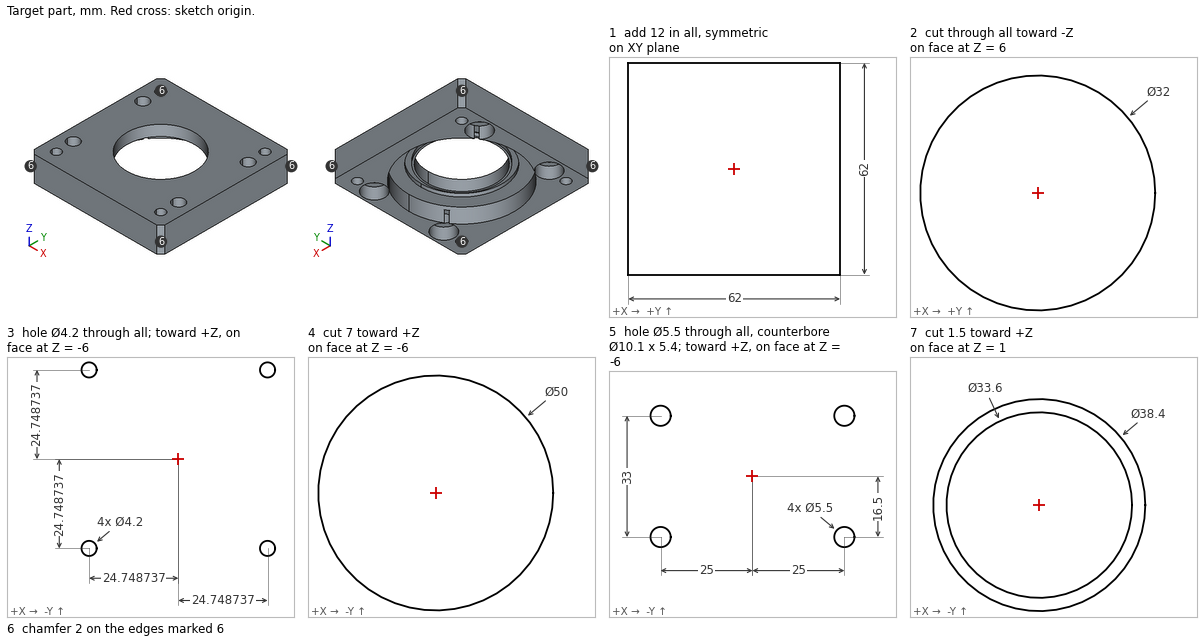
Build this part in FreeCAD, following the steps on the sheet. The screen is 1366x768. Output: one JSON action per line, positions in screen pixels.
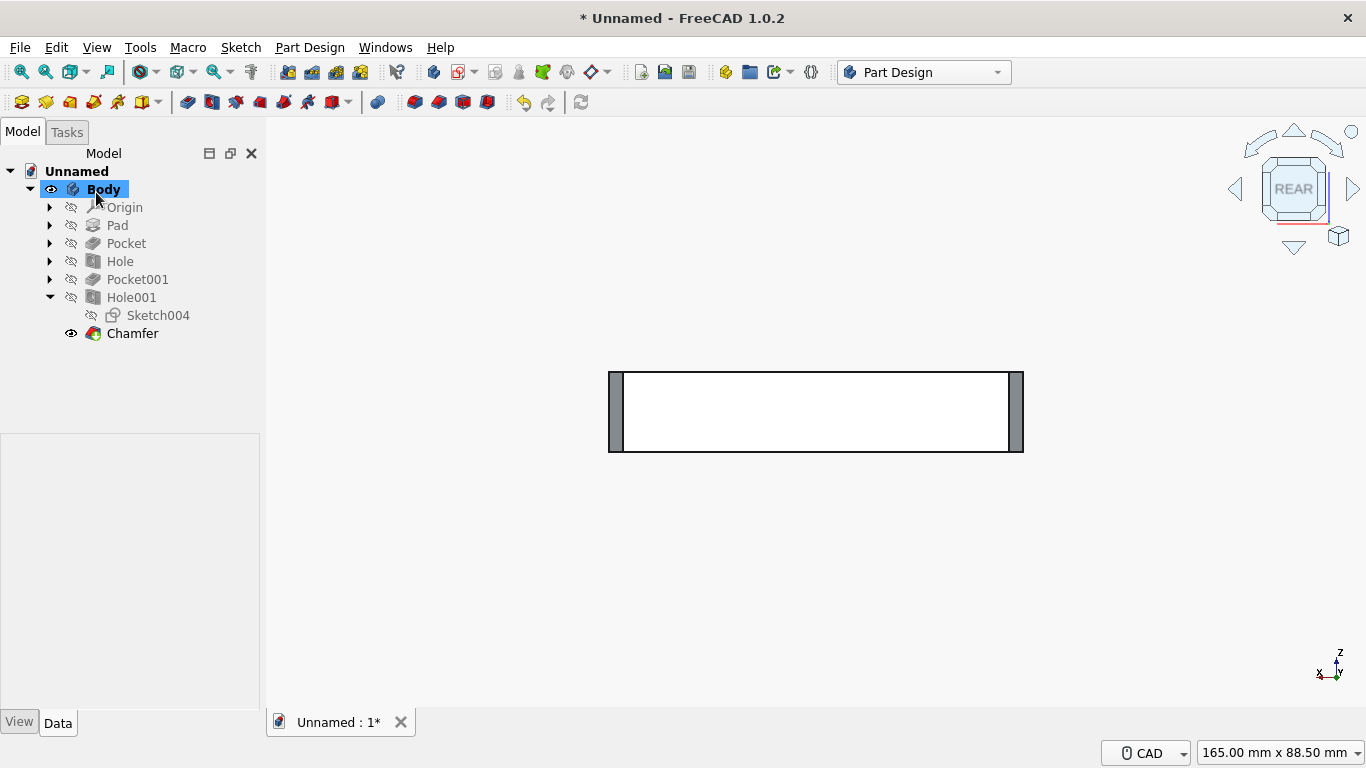
{"action": "left_click", "coordinate": [22, 72]}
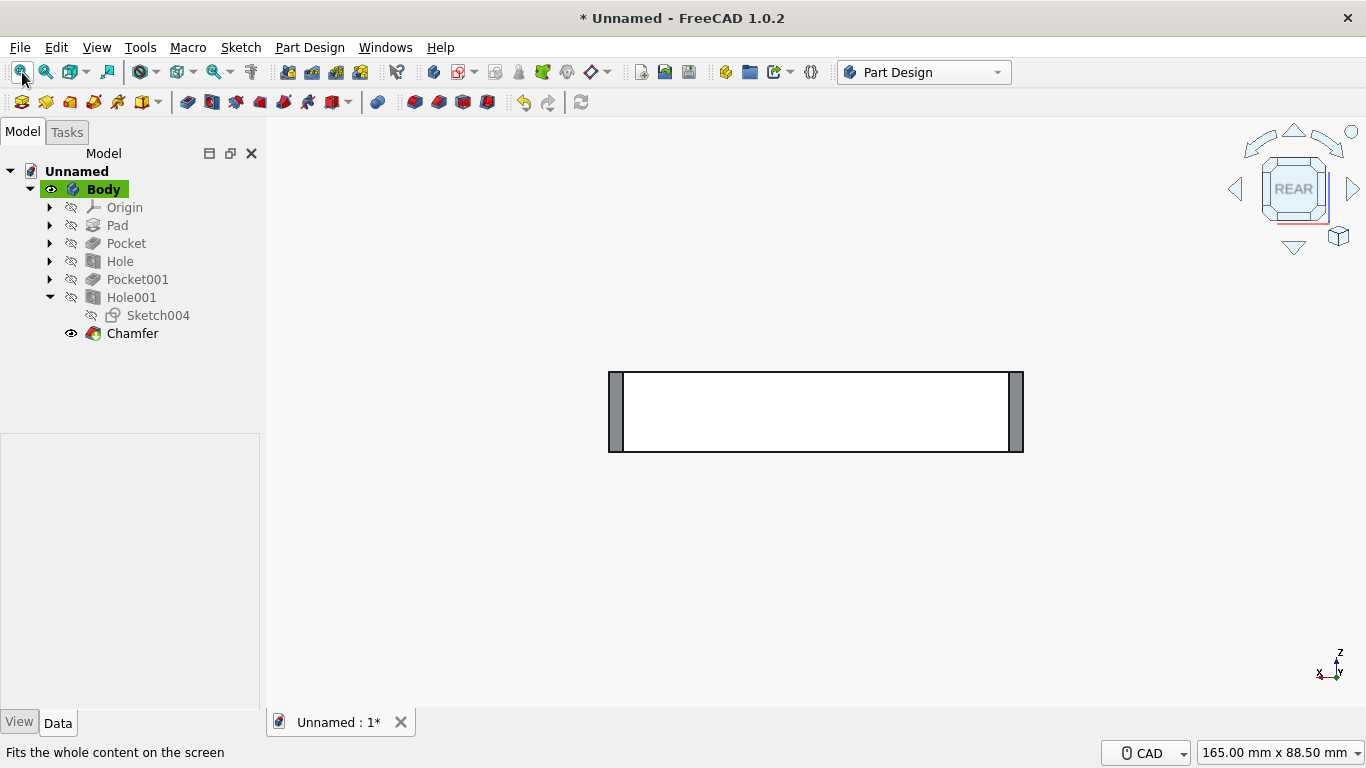
{"action": "key", "text": "5"}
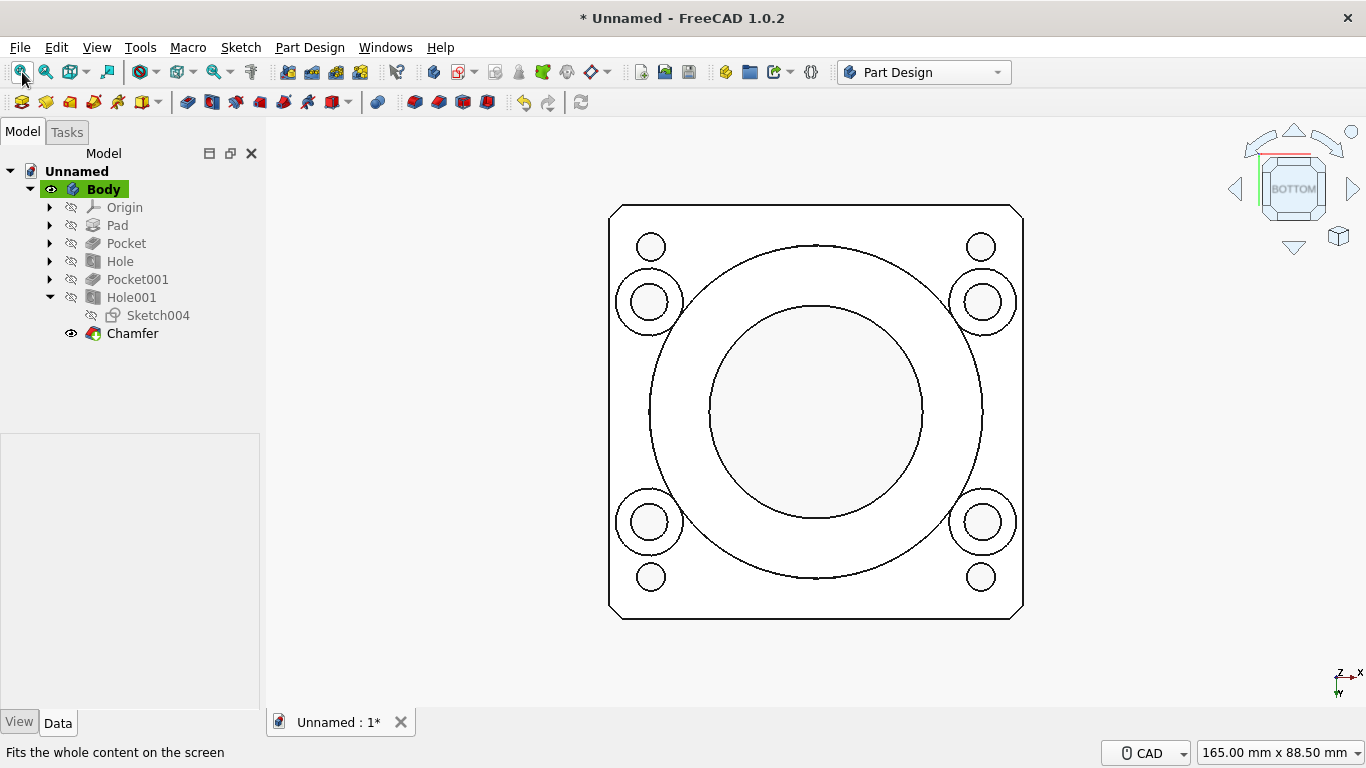
{"action": "left_click", "coordinate": [911, 316]}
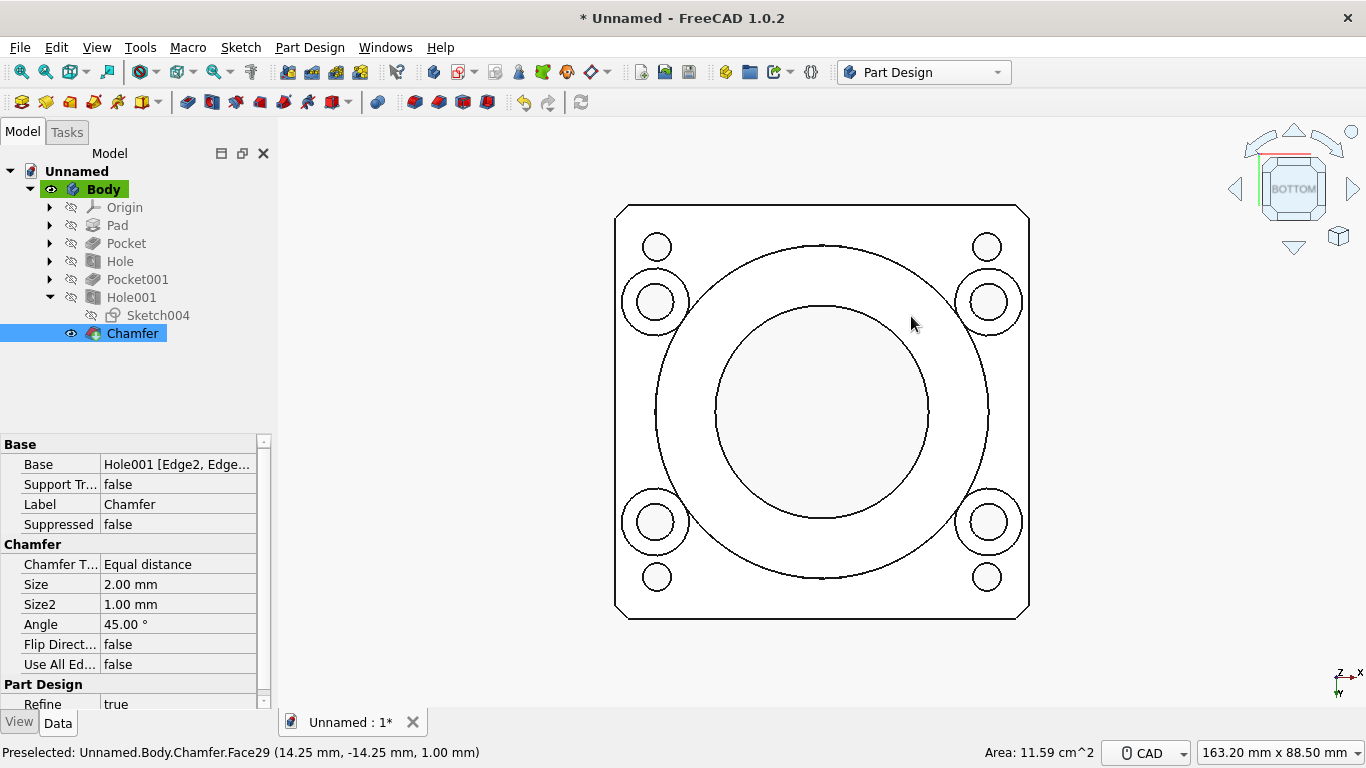
{"action": "left_click", "coordinate": [458, 72]}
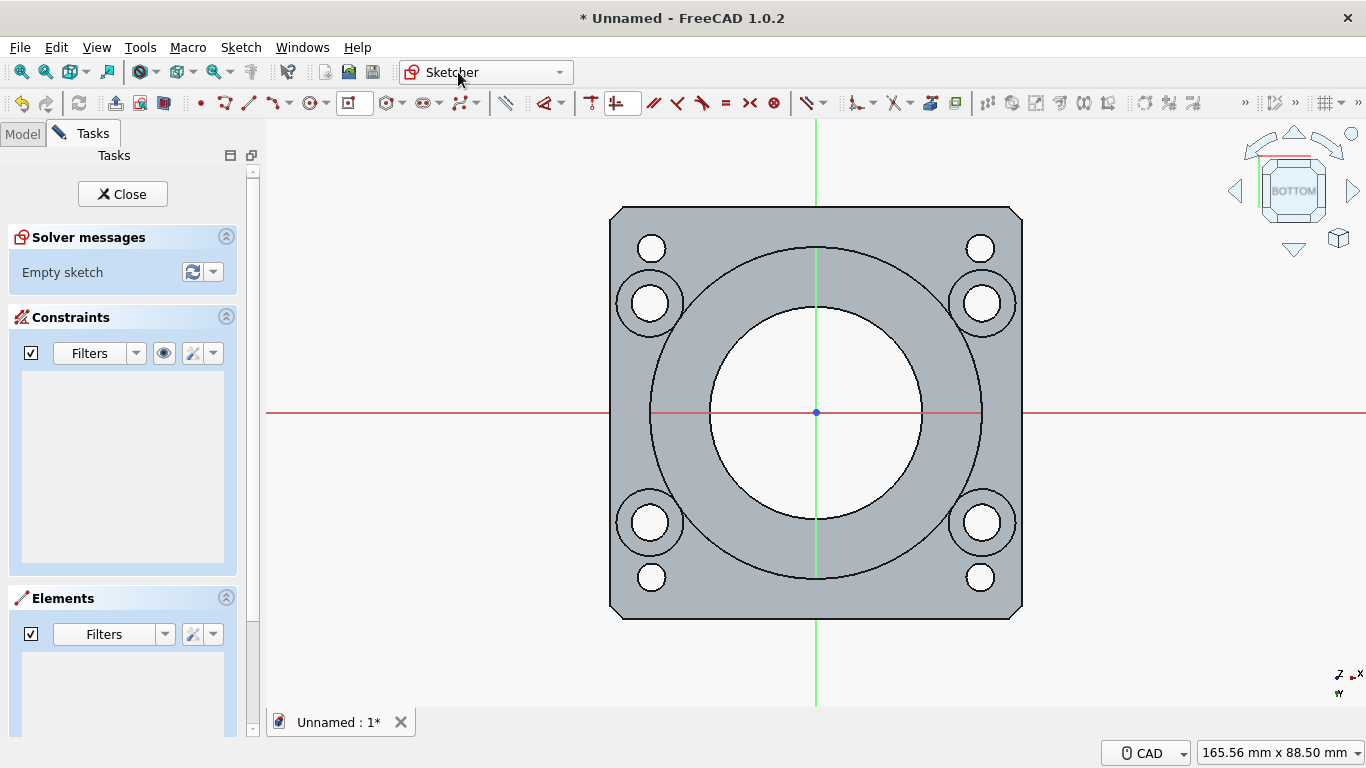
{"action": "scroll", "coordinate": [955, 413], "scroll_direction": "up", "scroll_amount": 2}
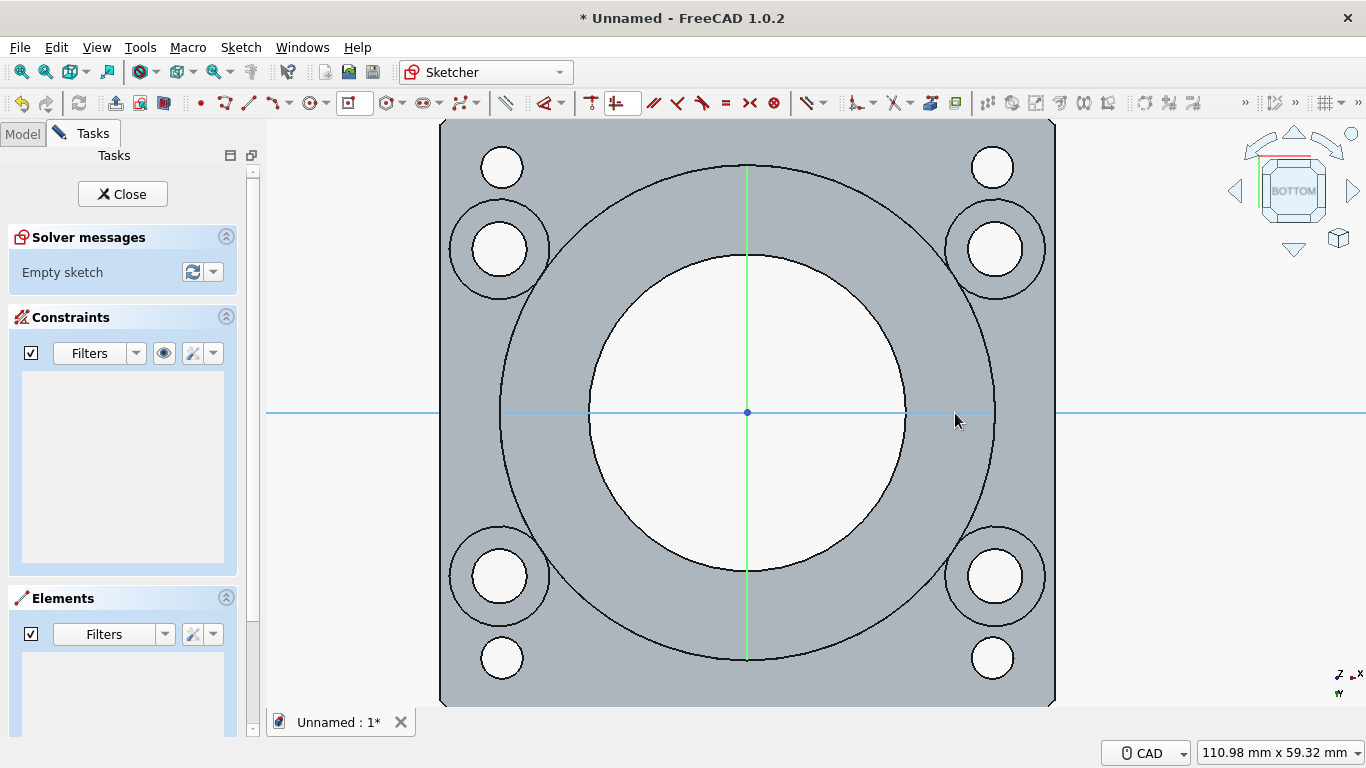
{"action": "left_click", "coordinate": [310, 104]}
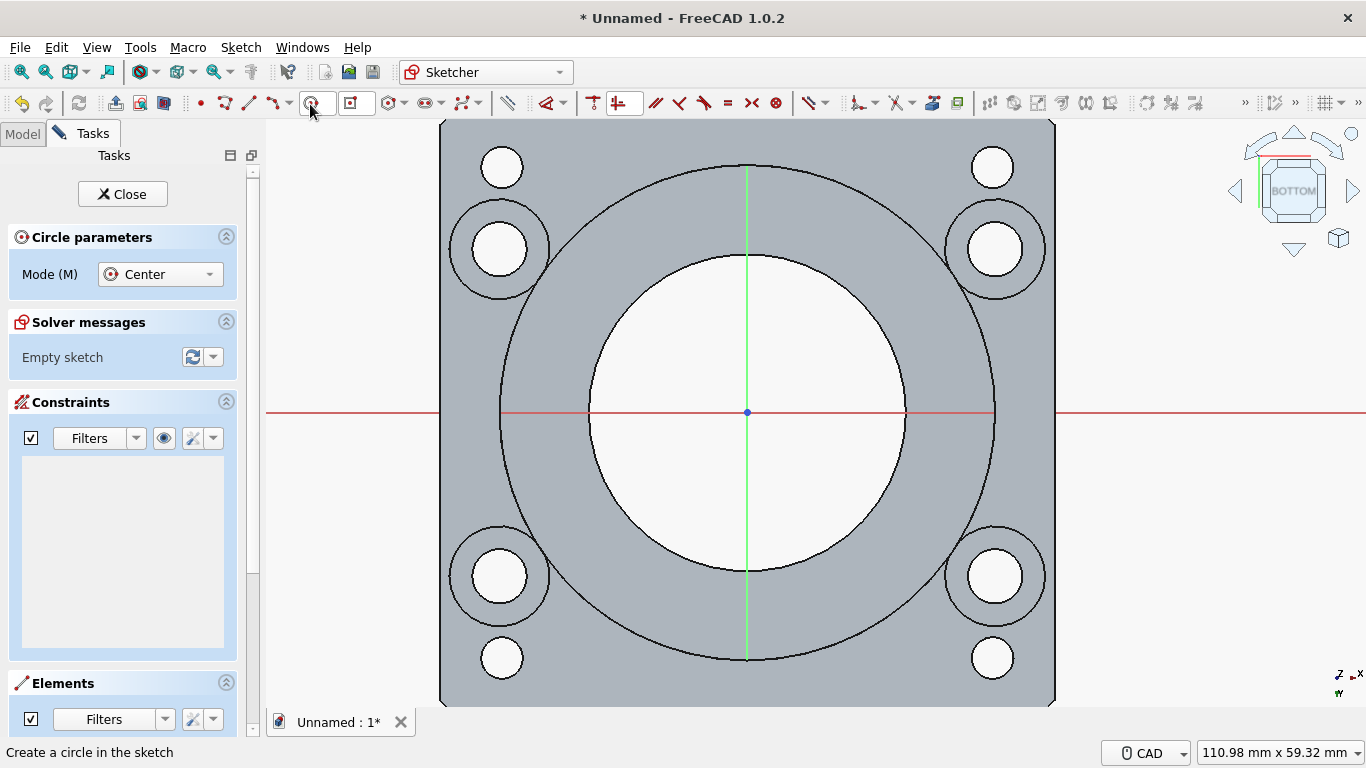
{"action": "left_click", "coordinate": [747, 413]}
{"action": "mouse_move", "coordinate": [882, 278]}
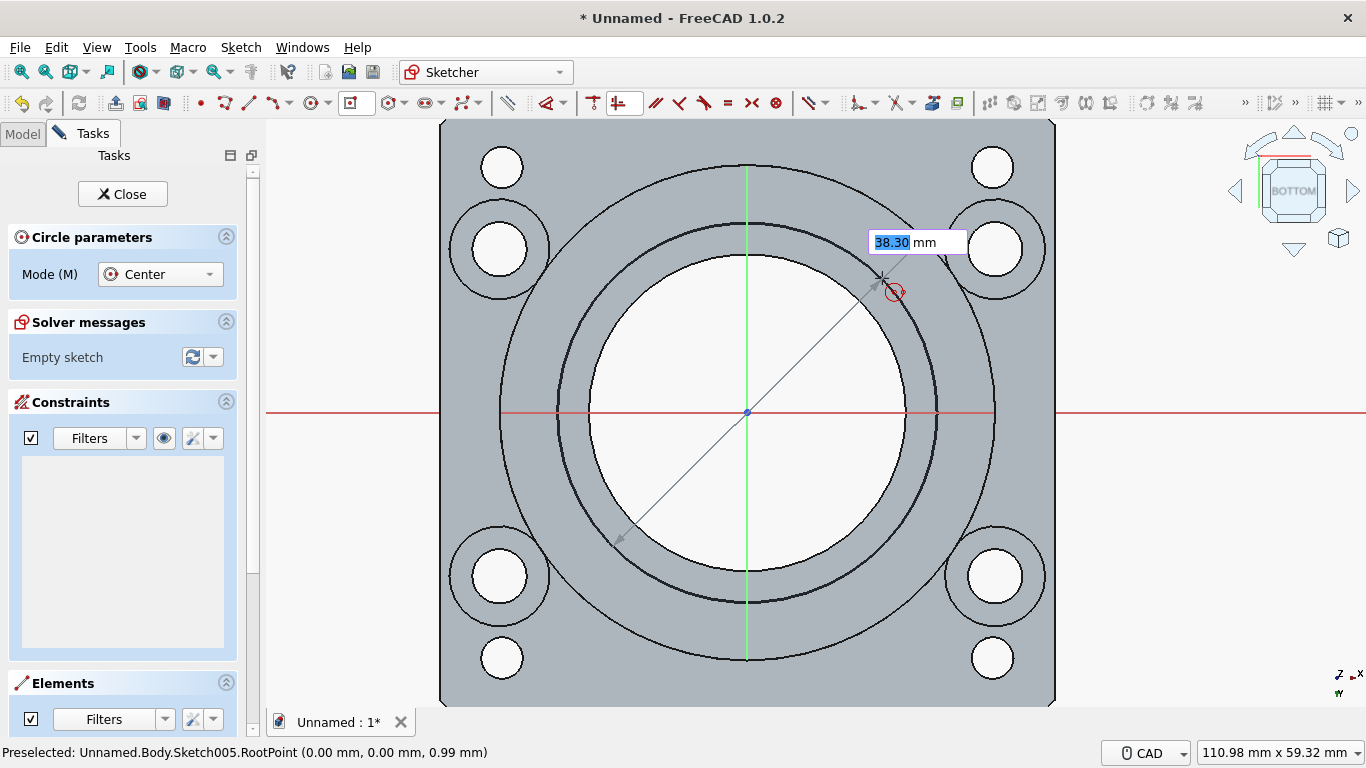
{"action": "type", "text": "38.4"}
{"action": "key", "text": "Return"}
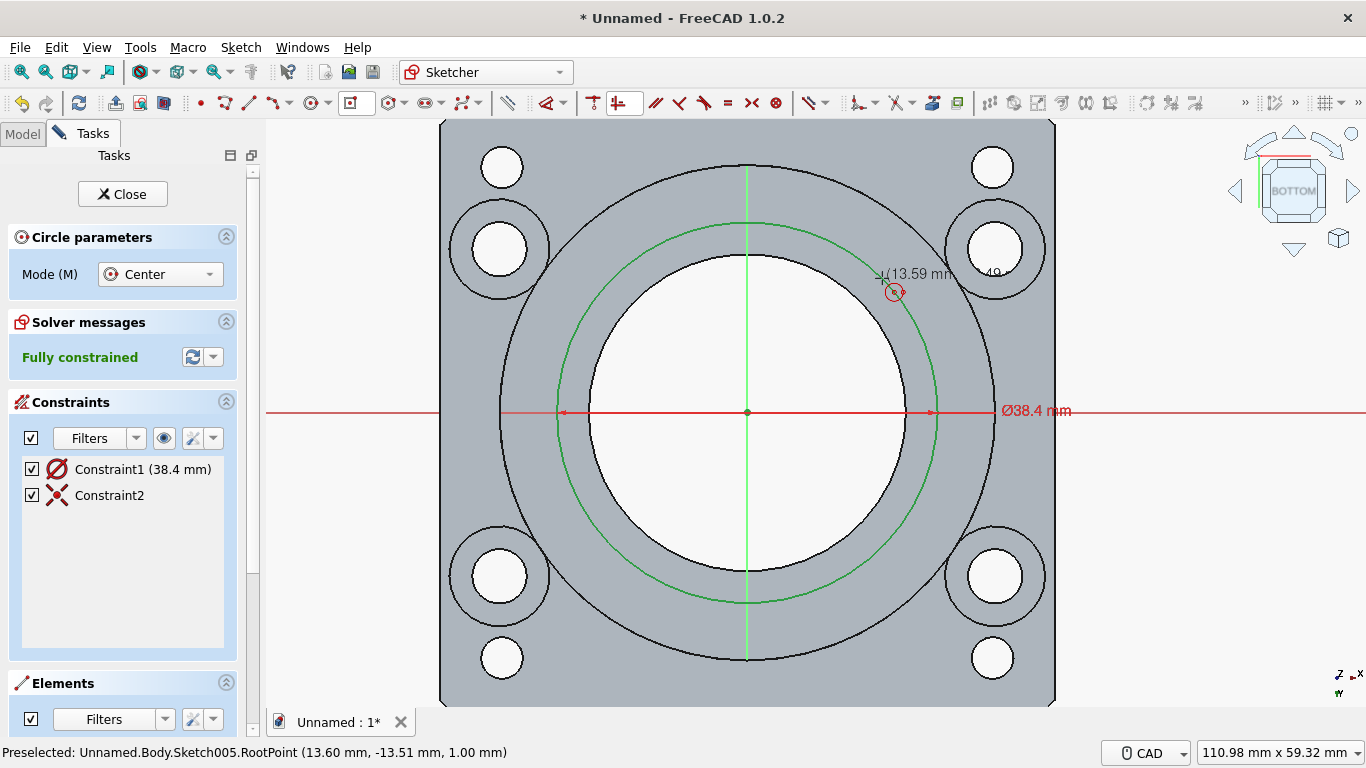
{"action": "left_click", "coordinate": [747, 413]}
{"action": "mouse_move", "coordinate": [865, 295]}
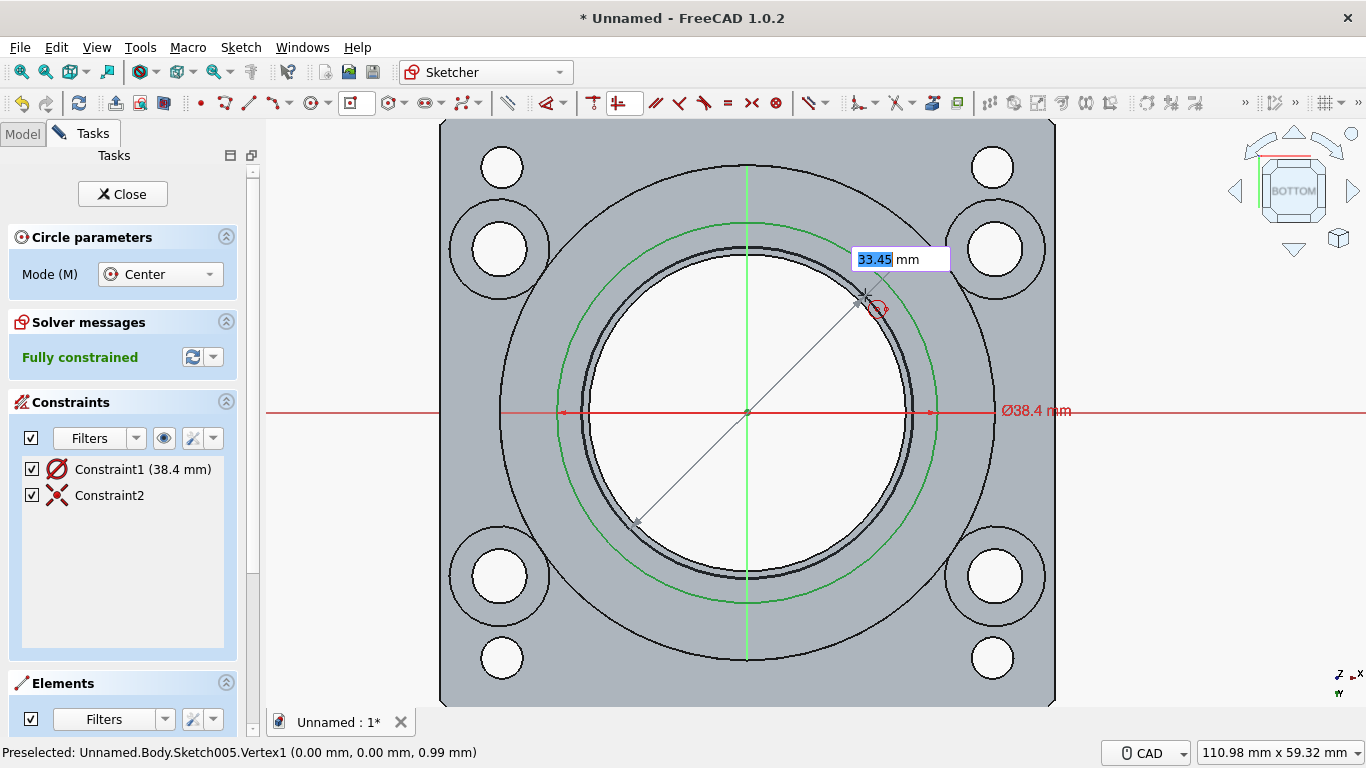
{"action": "type", "text": "33.6"}
{"action": "key", "text": "Return"}
{"action": "key", "text": "Escape"}